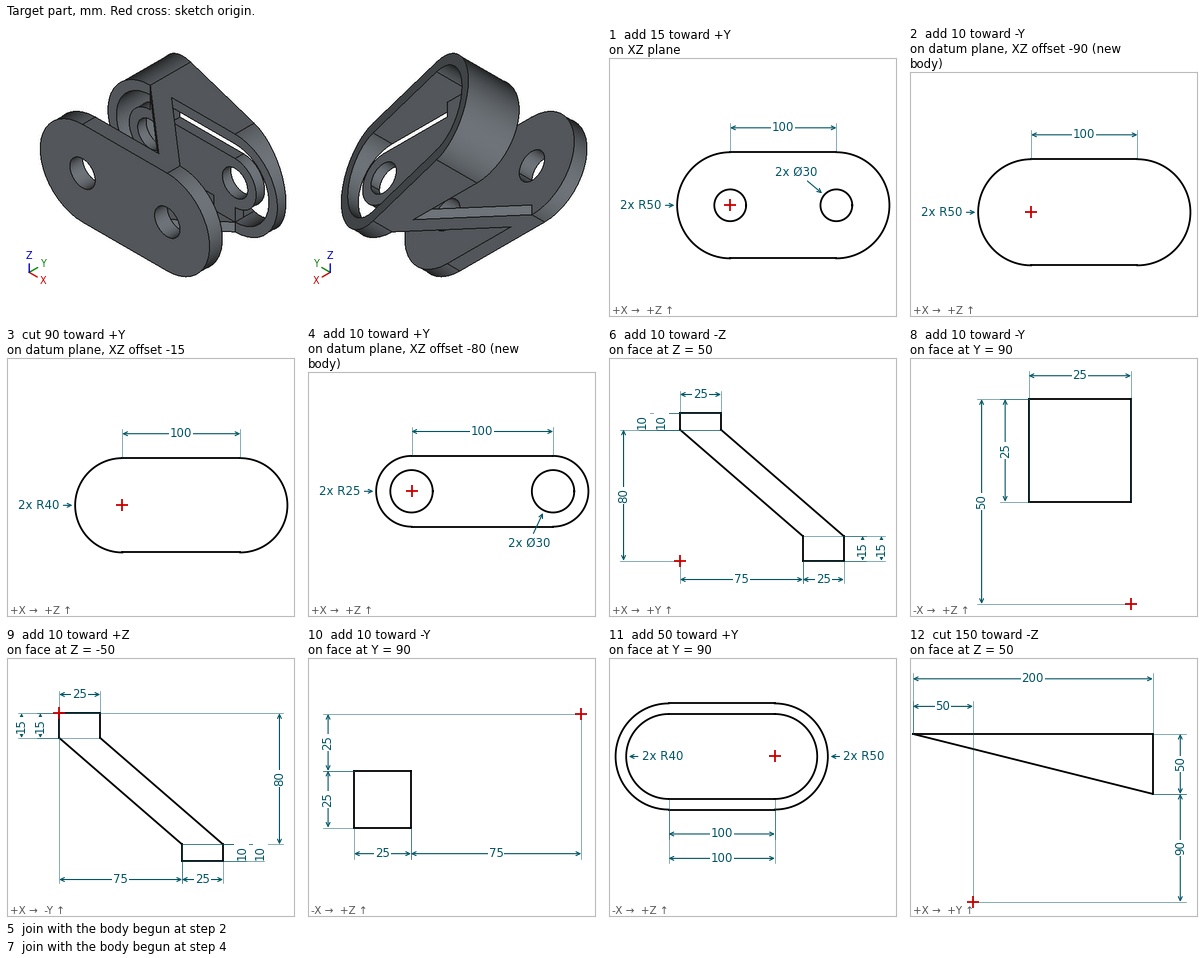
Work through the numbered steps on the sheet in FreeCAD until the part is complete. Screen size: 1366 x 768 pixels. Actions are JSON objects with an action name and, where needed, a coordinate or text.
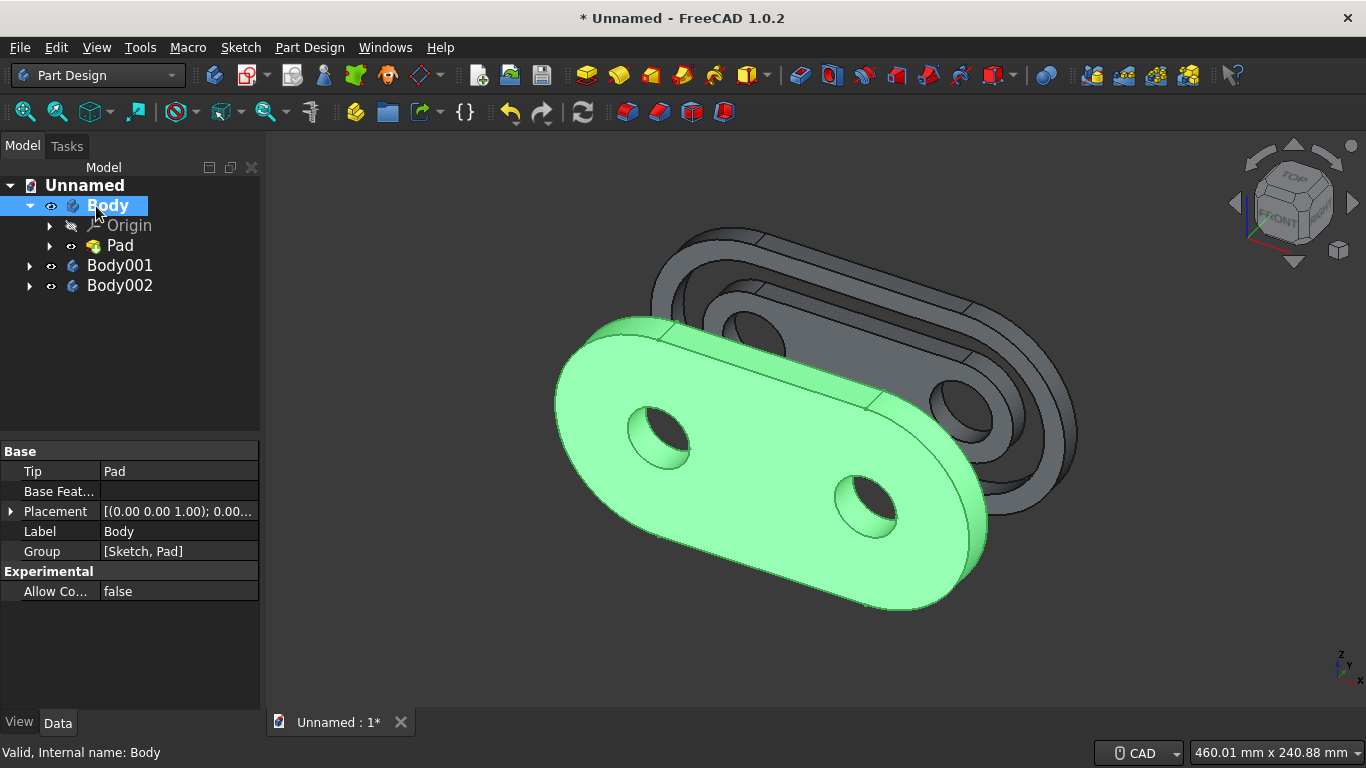
{"action": "left_click", "coordinate": [146, 591]}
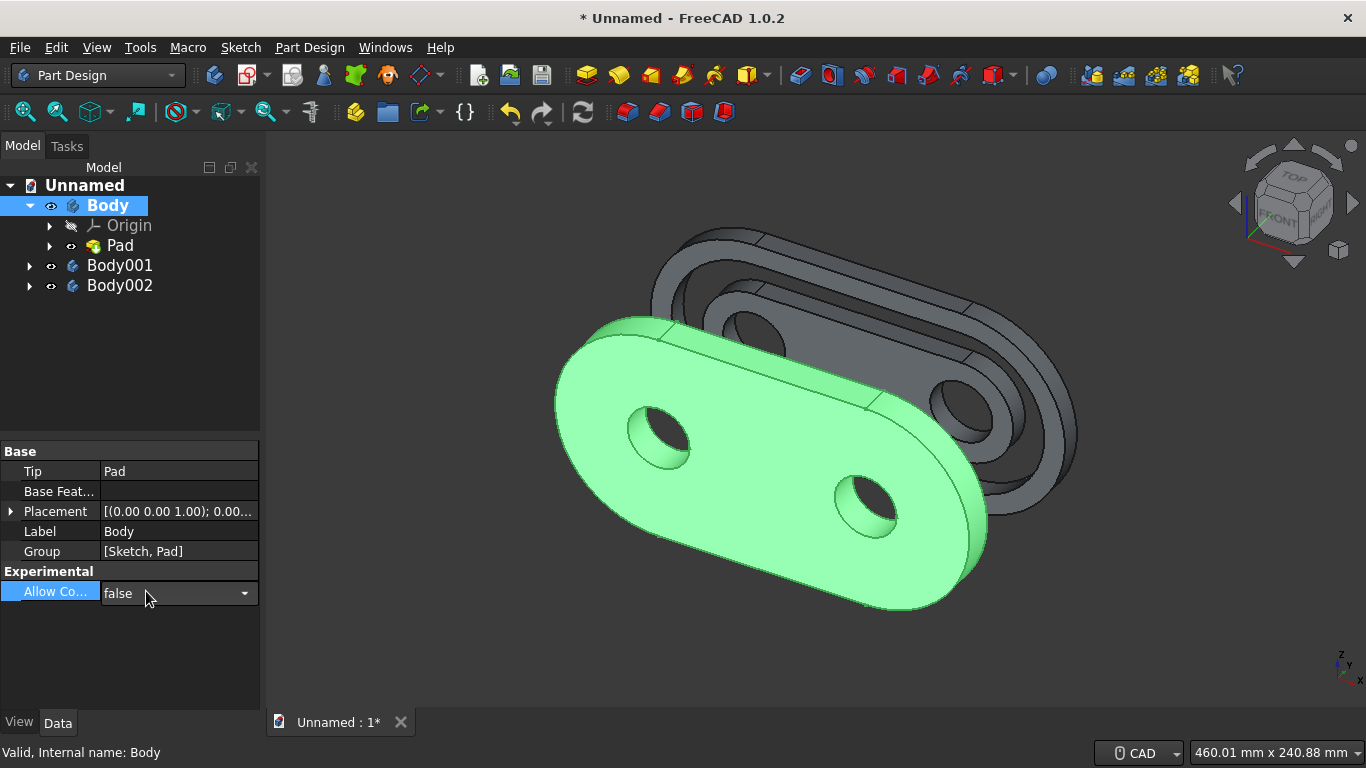
{"action": "left_click", "coordinate": [146, 591]}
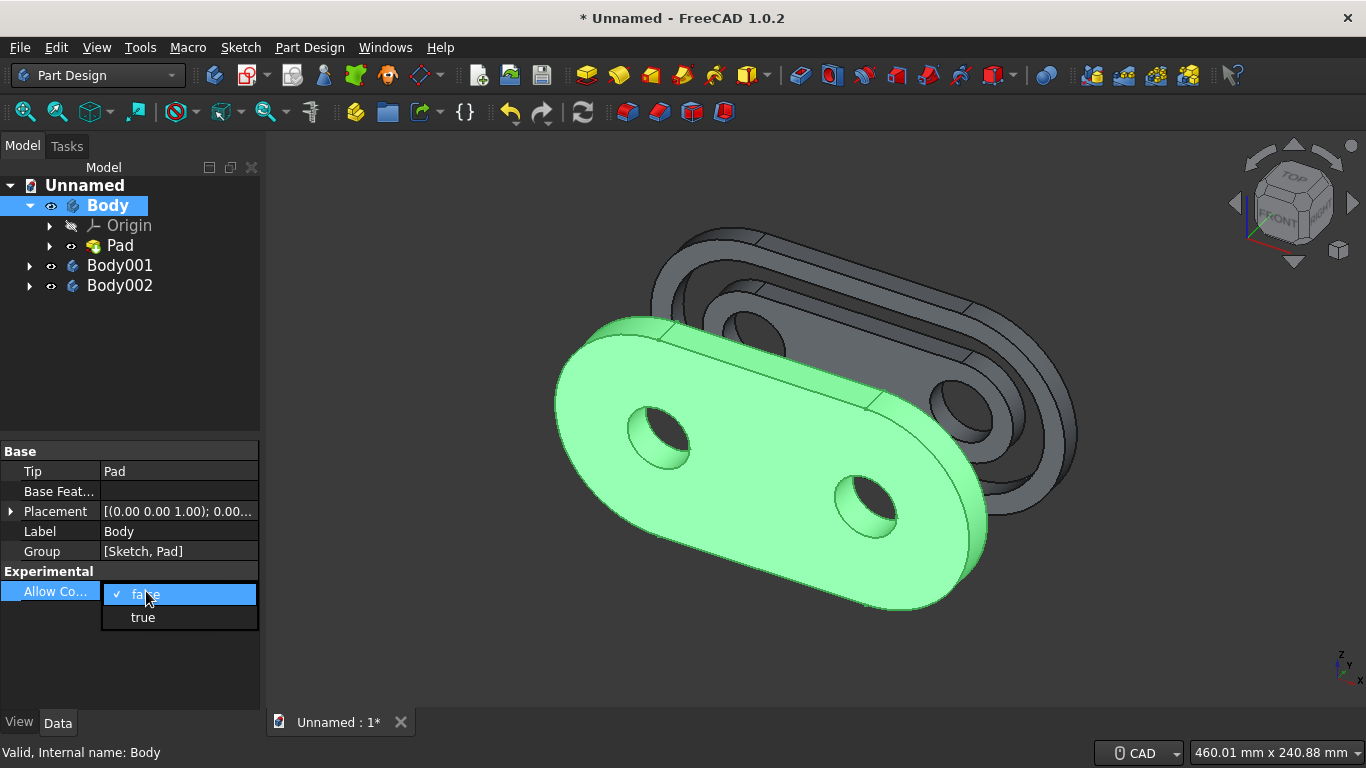
{"action": "left_click", "coordinate": [179, 618]}
{"action": "key", "text": "Return"}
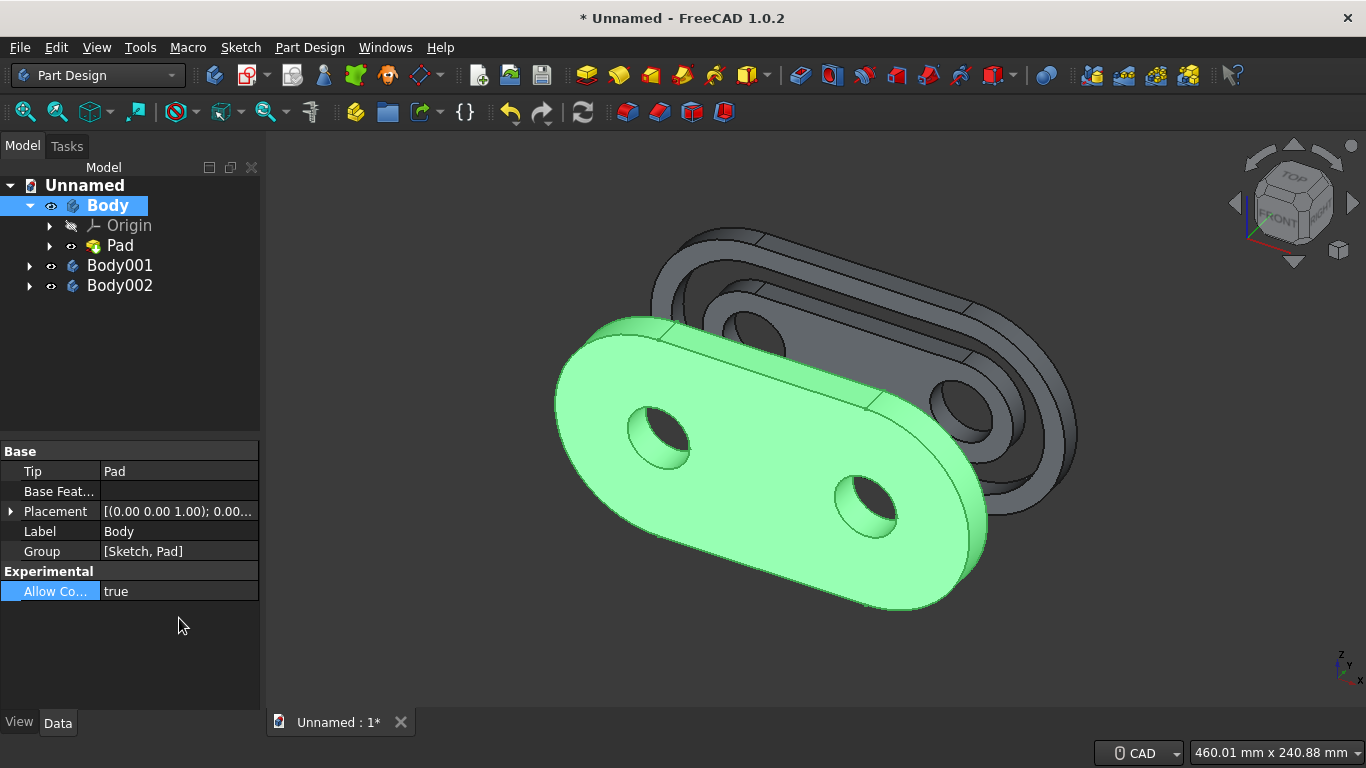
{"action": "left_click", "coordinate": [96, 266]}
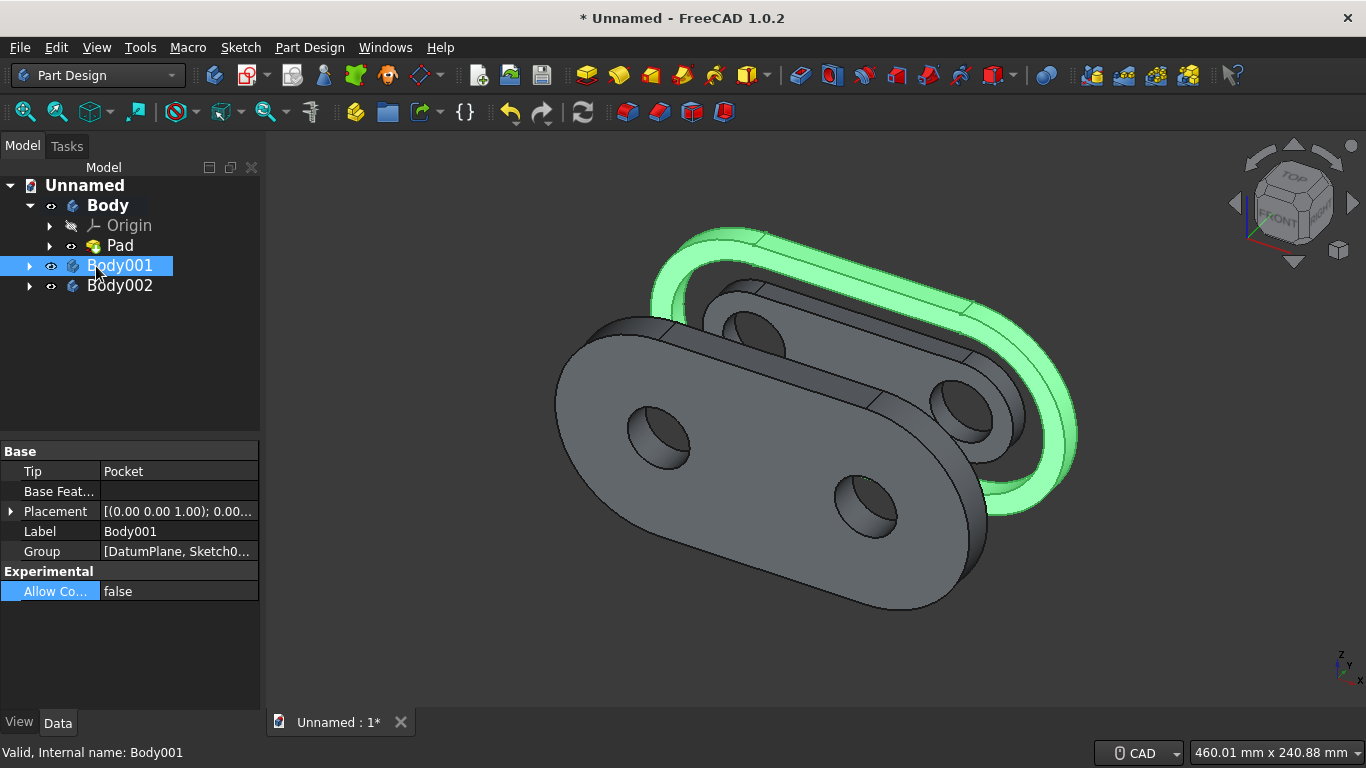
{"action": "left_click", "coordinate": [1048, 76]}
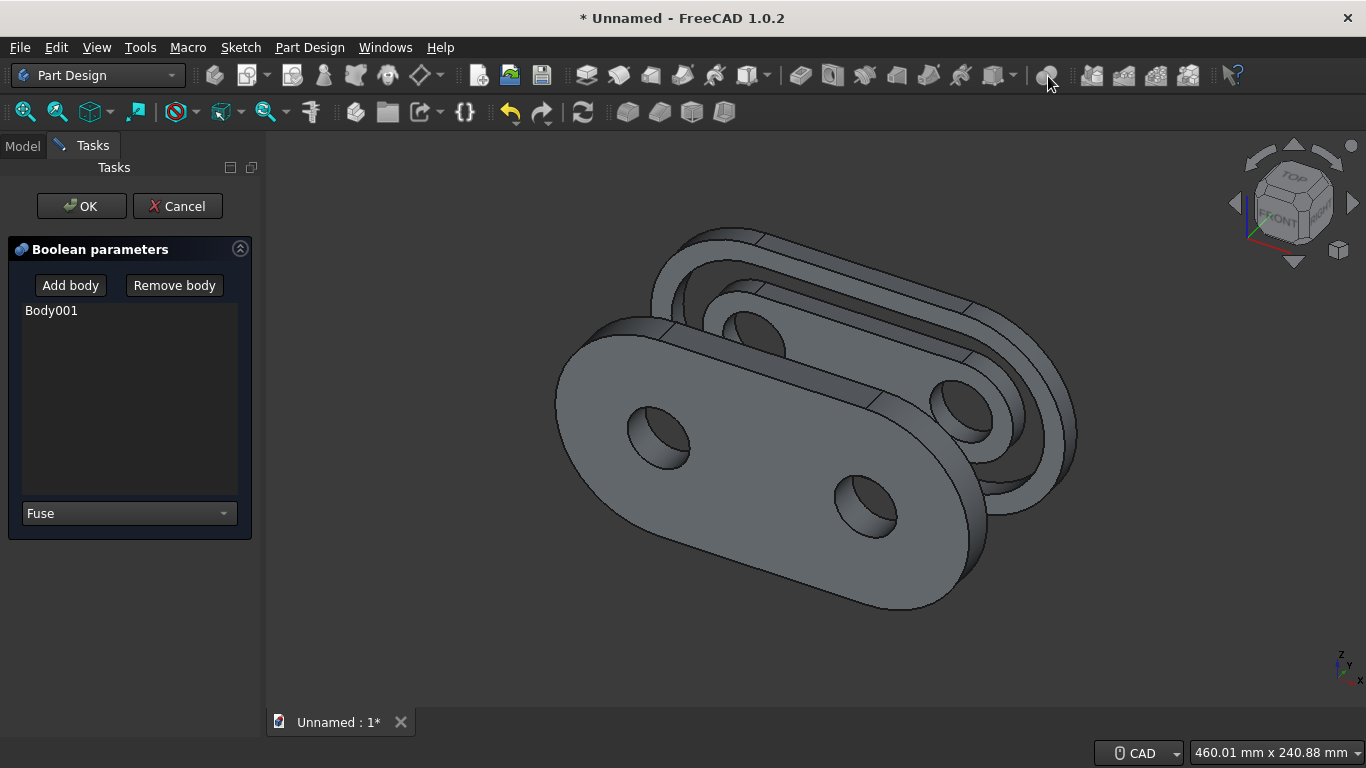
{"action": "left_click", "coordinate": [82, 206]}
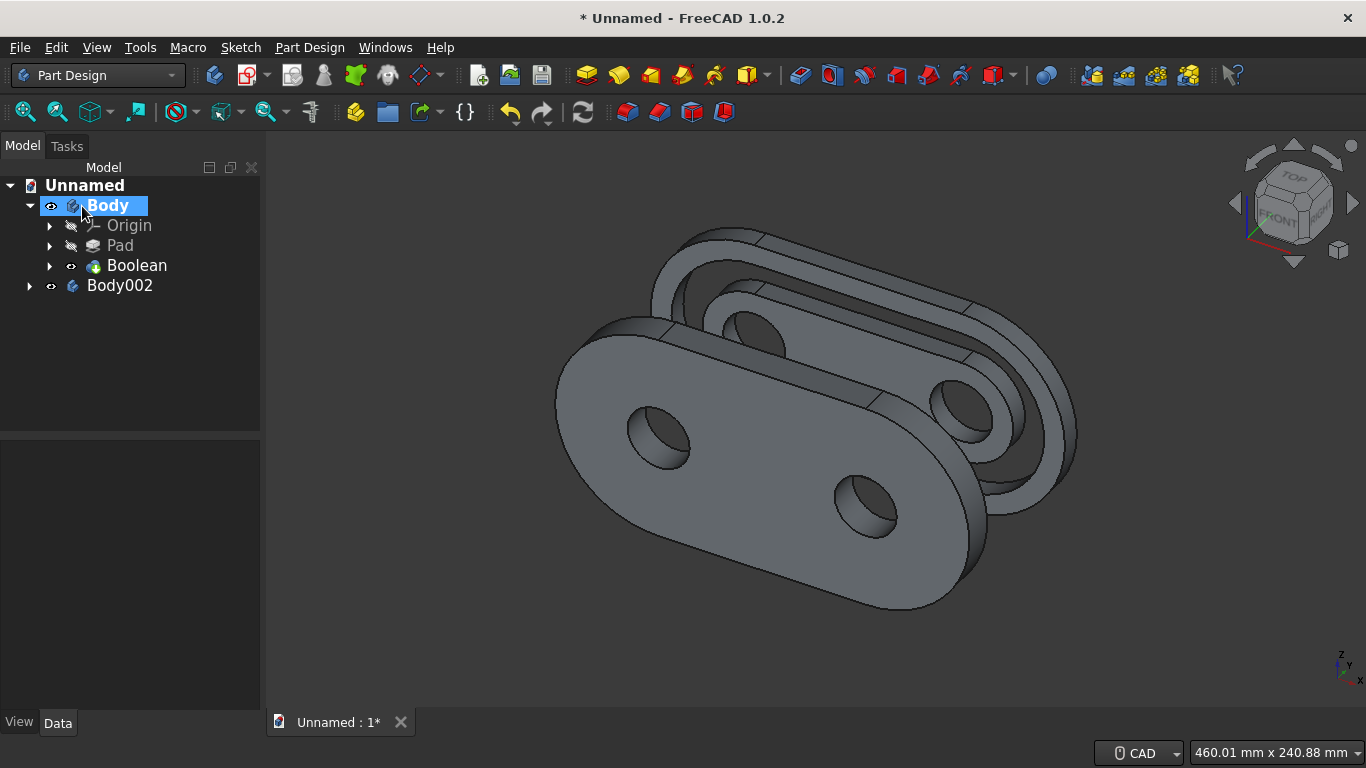
{"action": "left_click", "coordinate": [830, 384]}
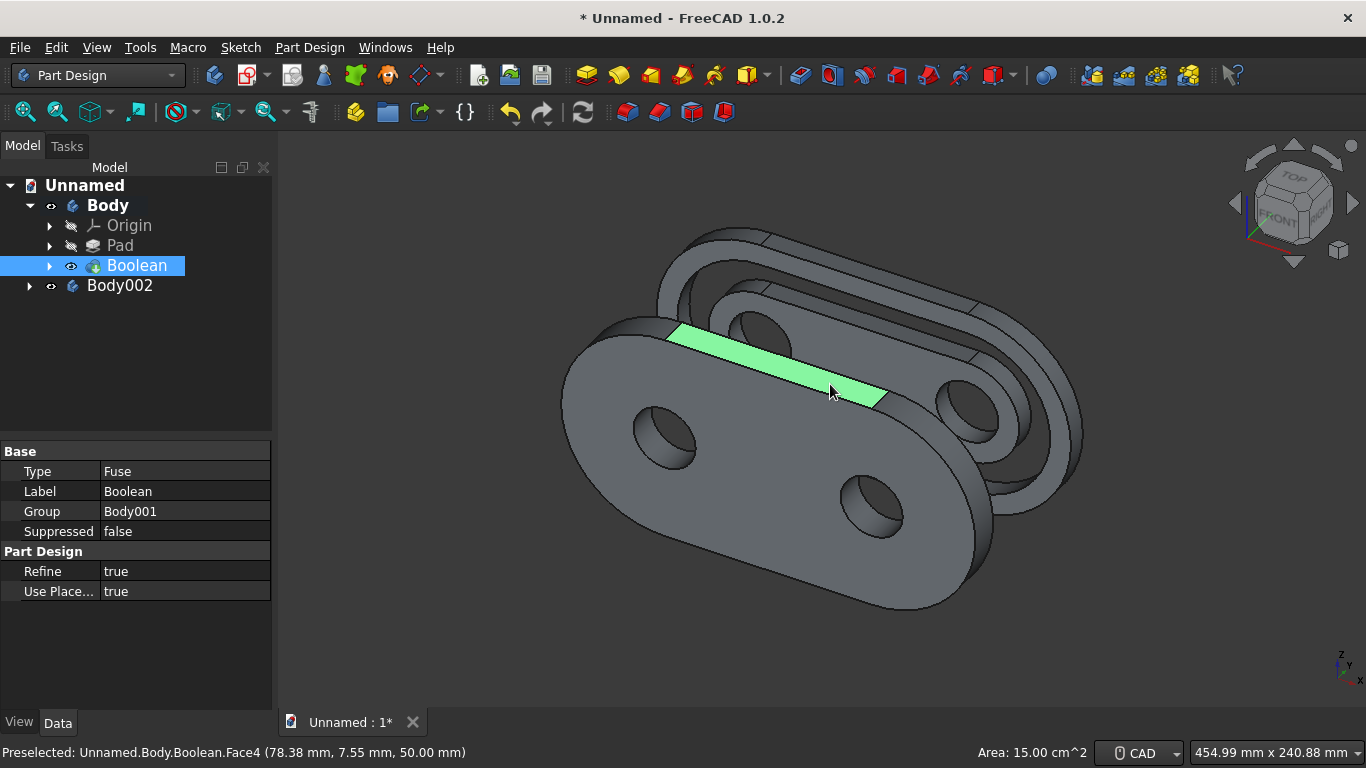
{"action": "left_click", "coordinate": [248, 76]}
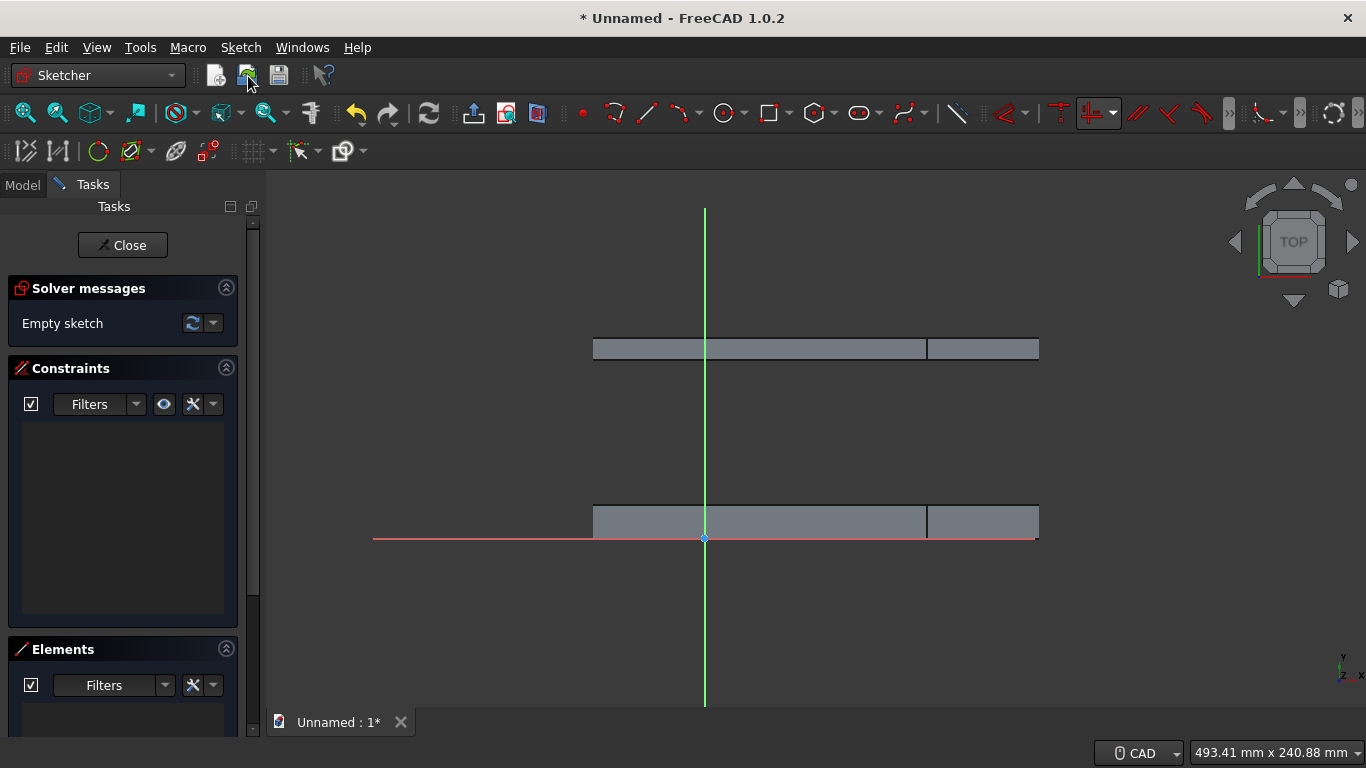
{"action": "scroll", "coordinate": [899, 438], "scroll_direction": "up", "scroll_amount": 3}